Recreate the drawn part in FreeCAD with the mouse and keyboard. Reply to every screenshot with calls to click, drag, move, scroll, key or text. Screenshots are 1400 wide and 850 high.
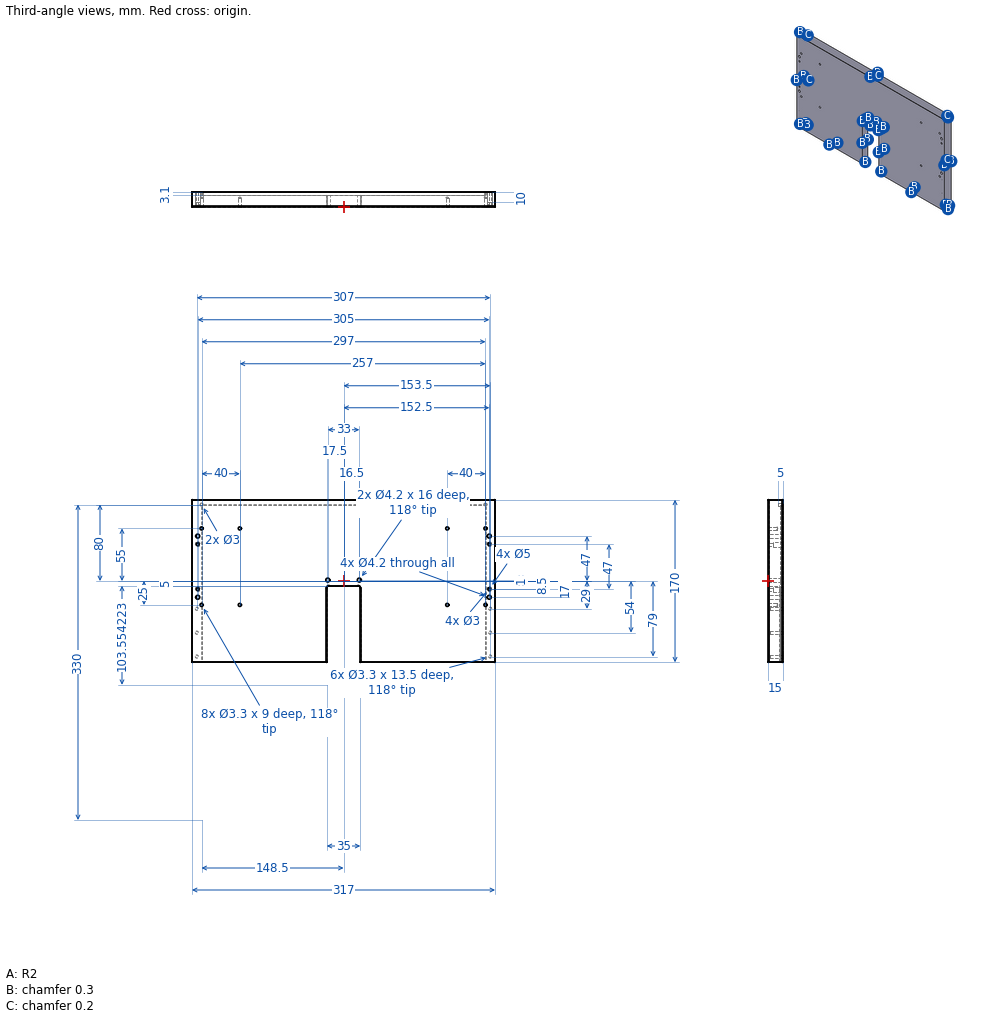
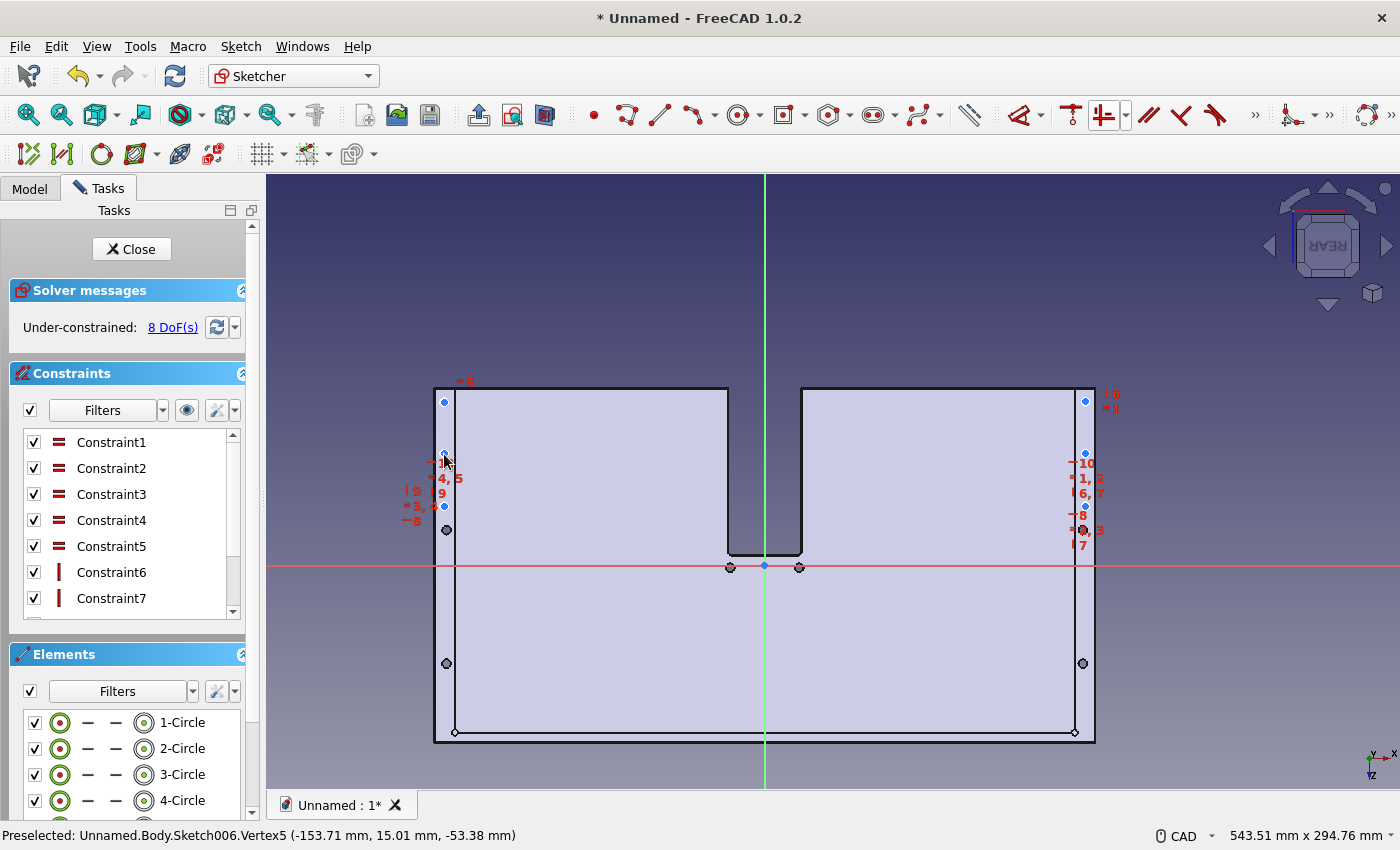
click(444, 453)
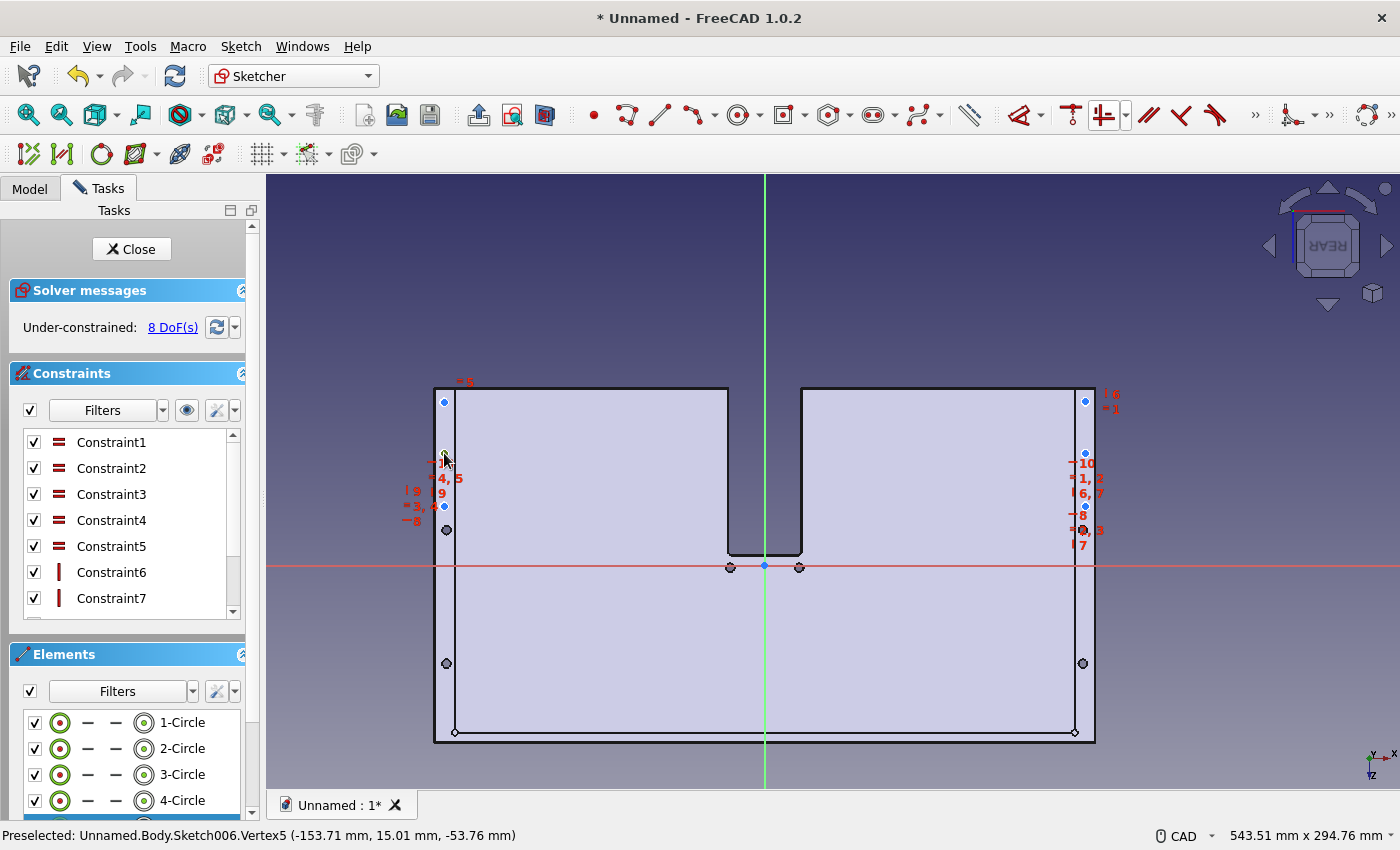
click(444, 402)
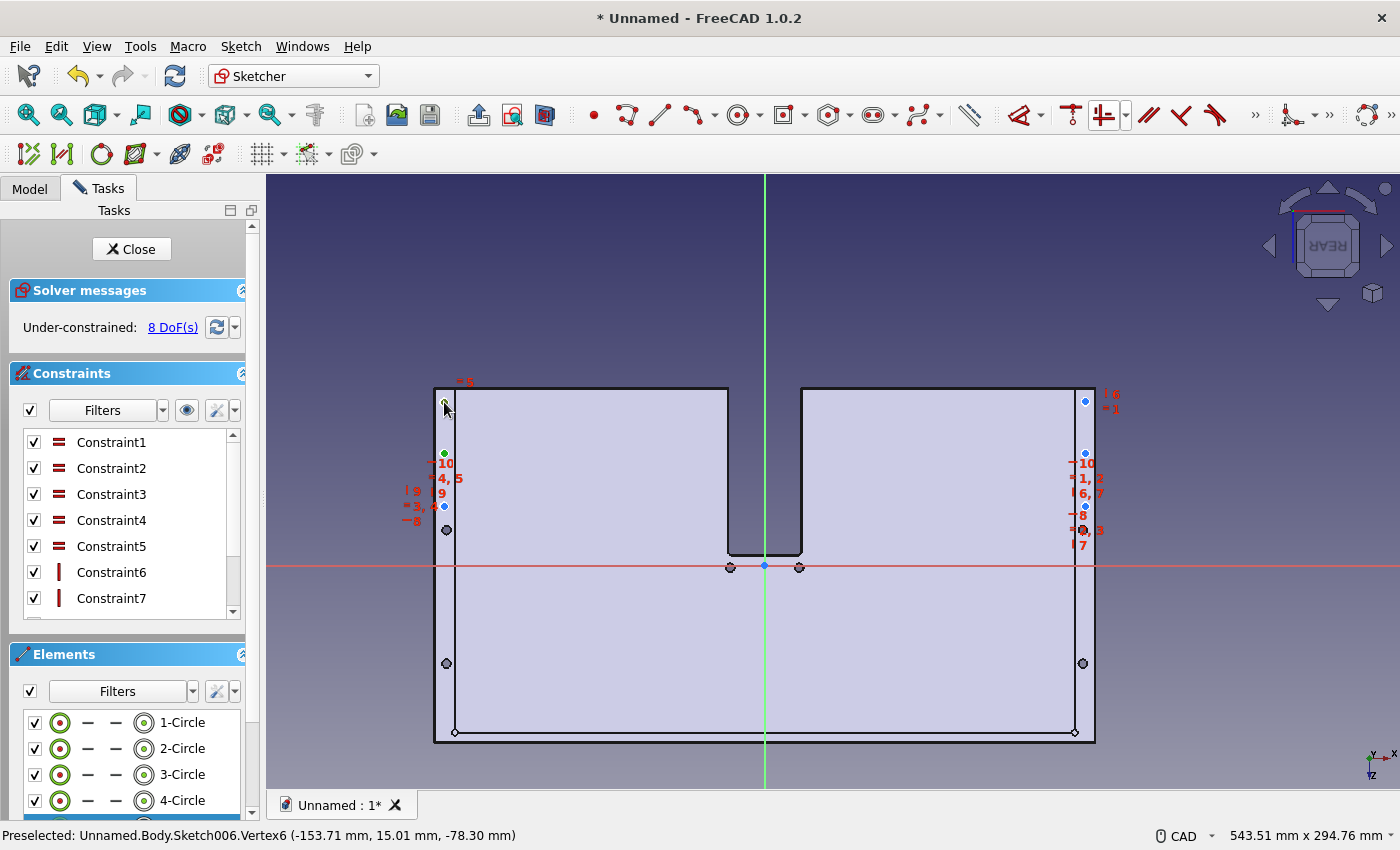
key(v)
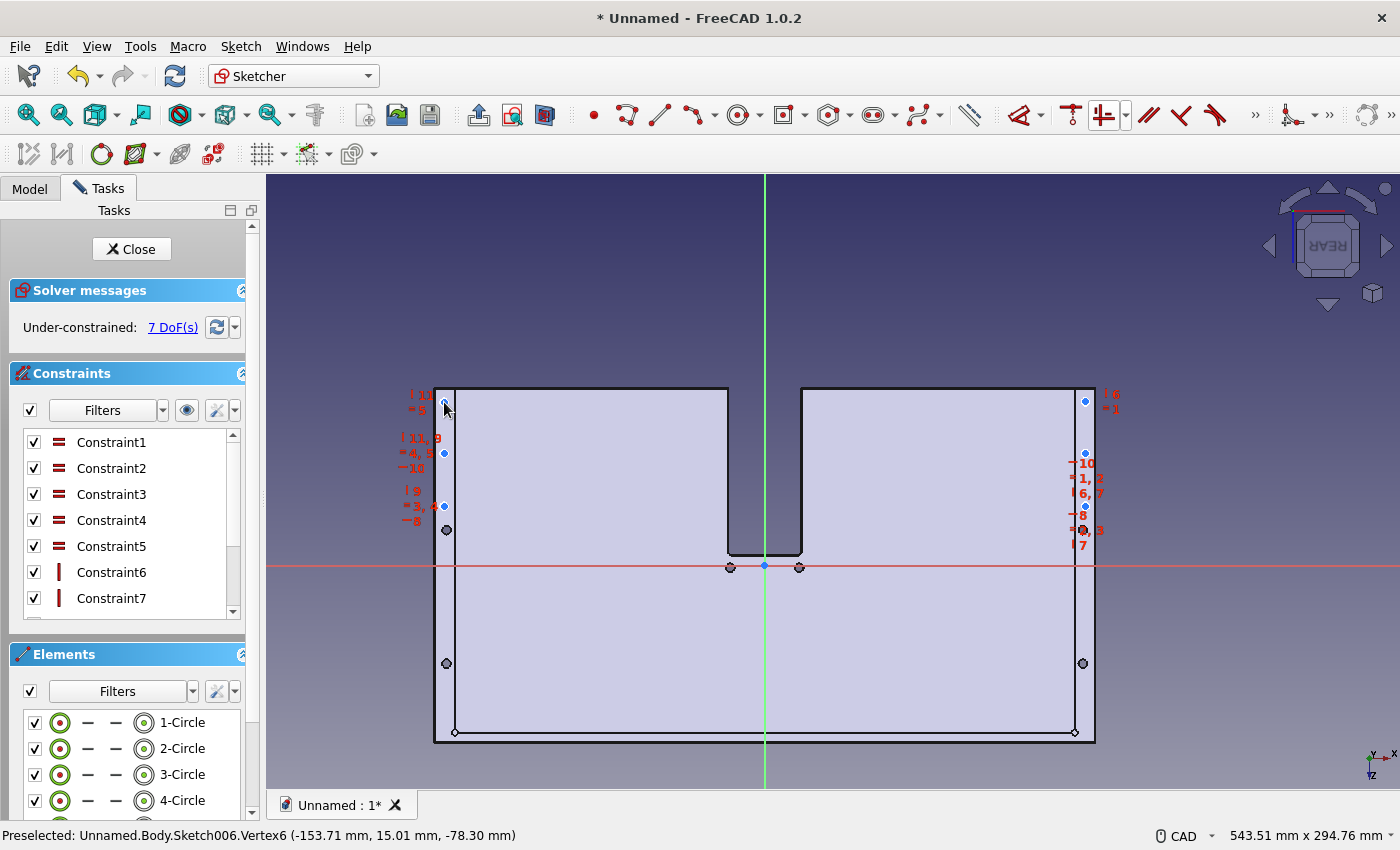
click(1085, 402)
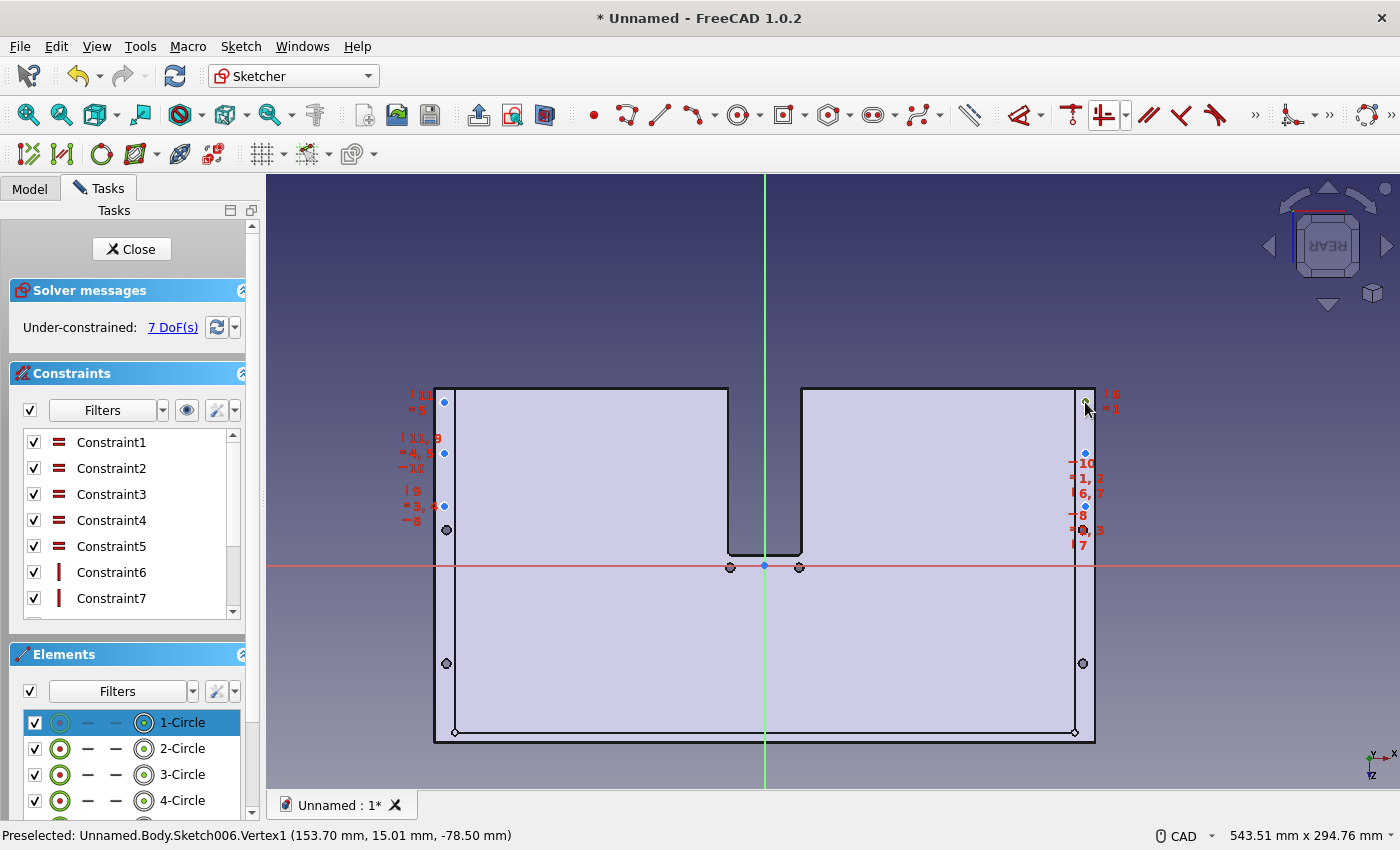
click(444, 402)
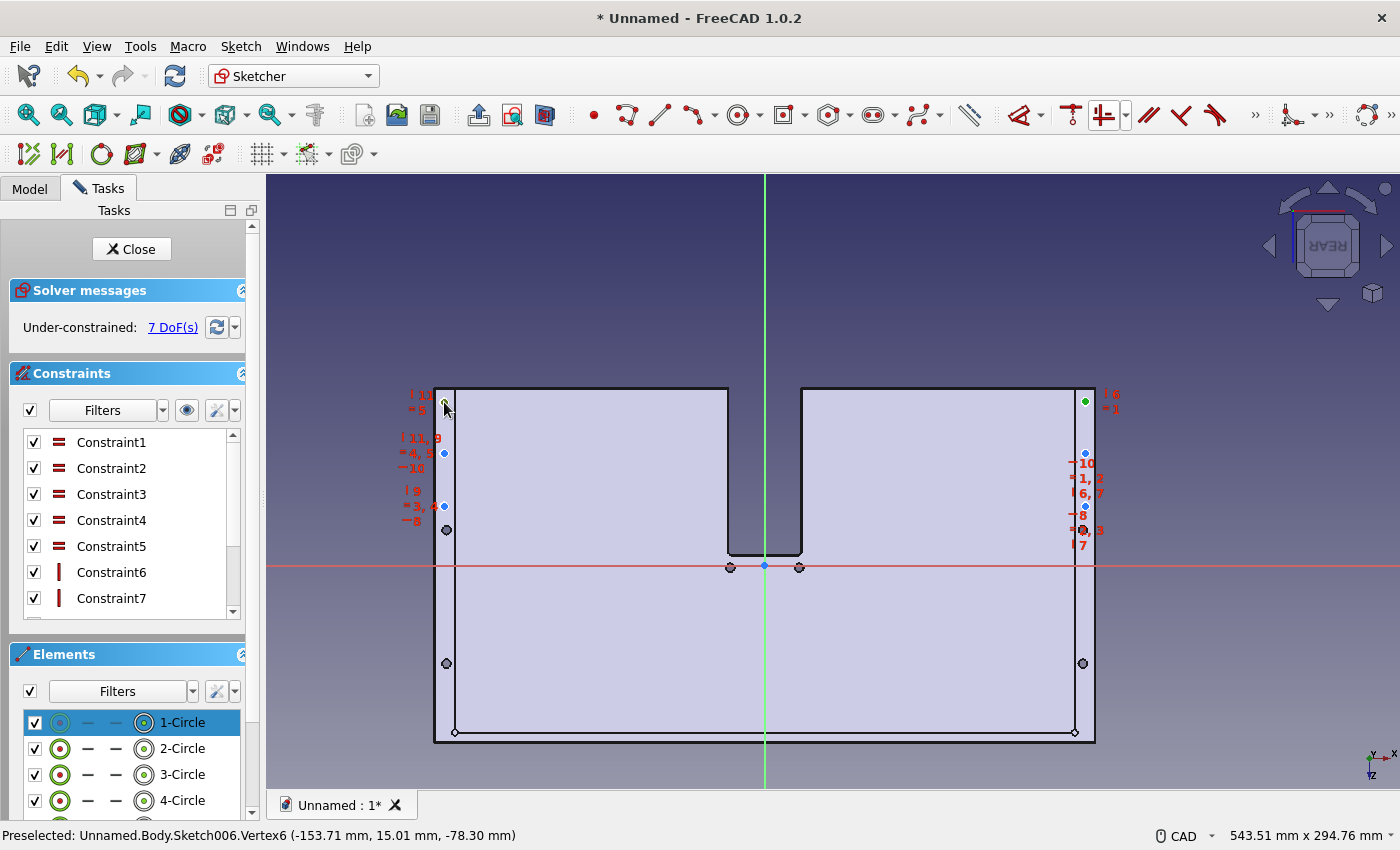
key(h)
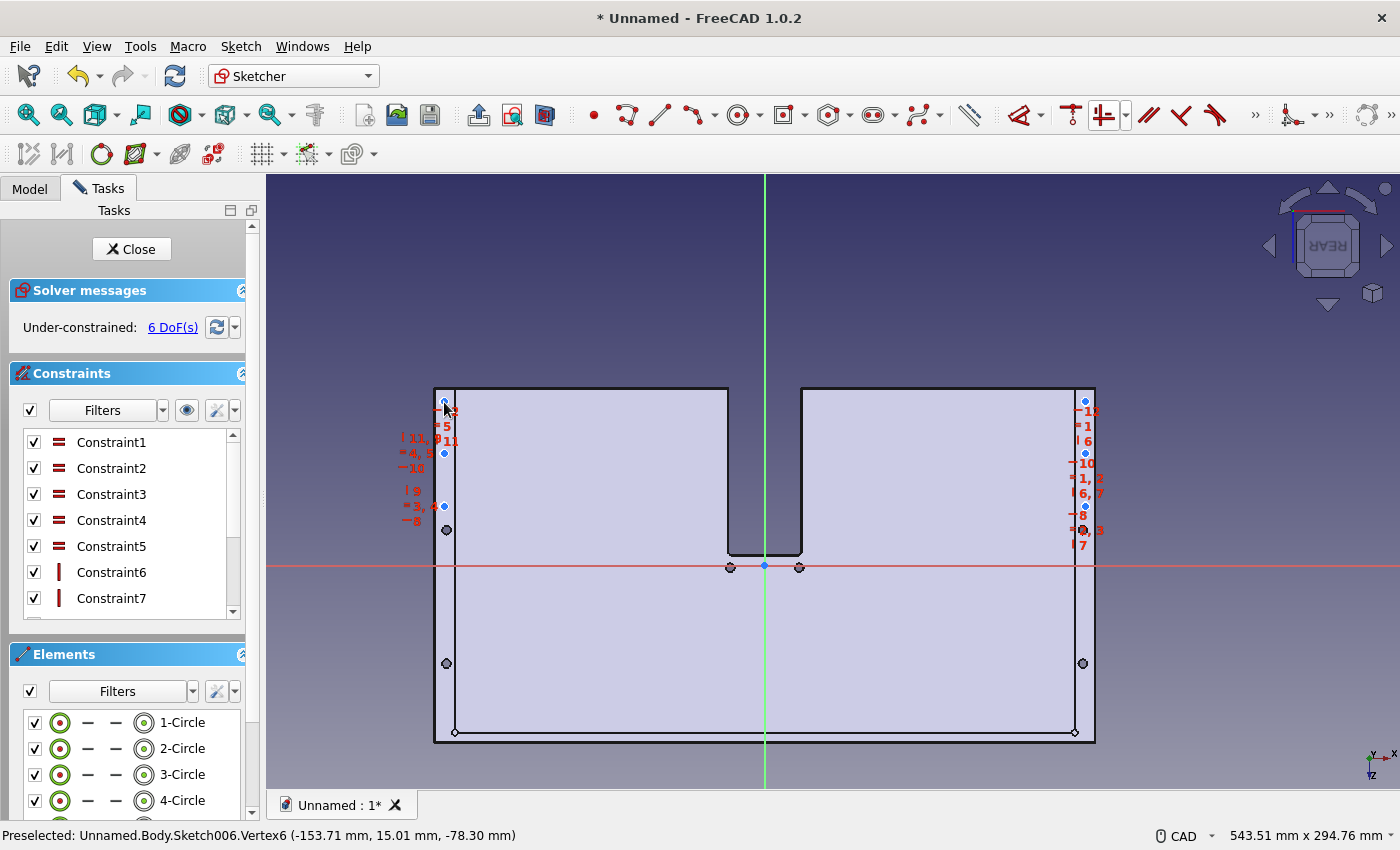
click(1018, 116)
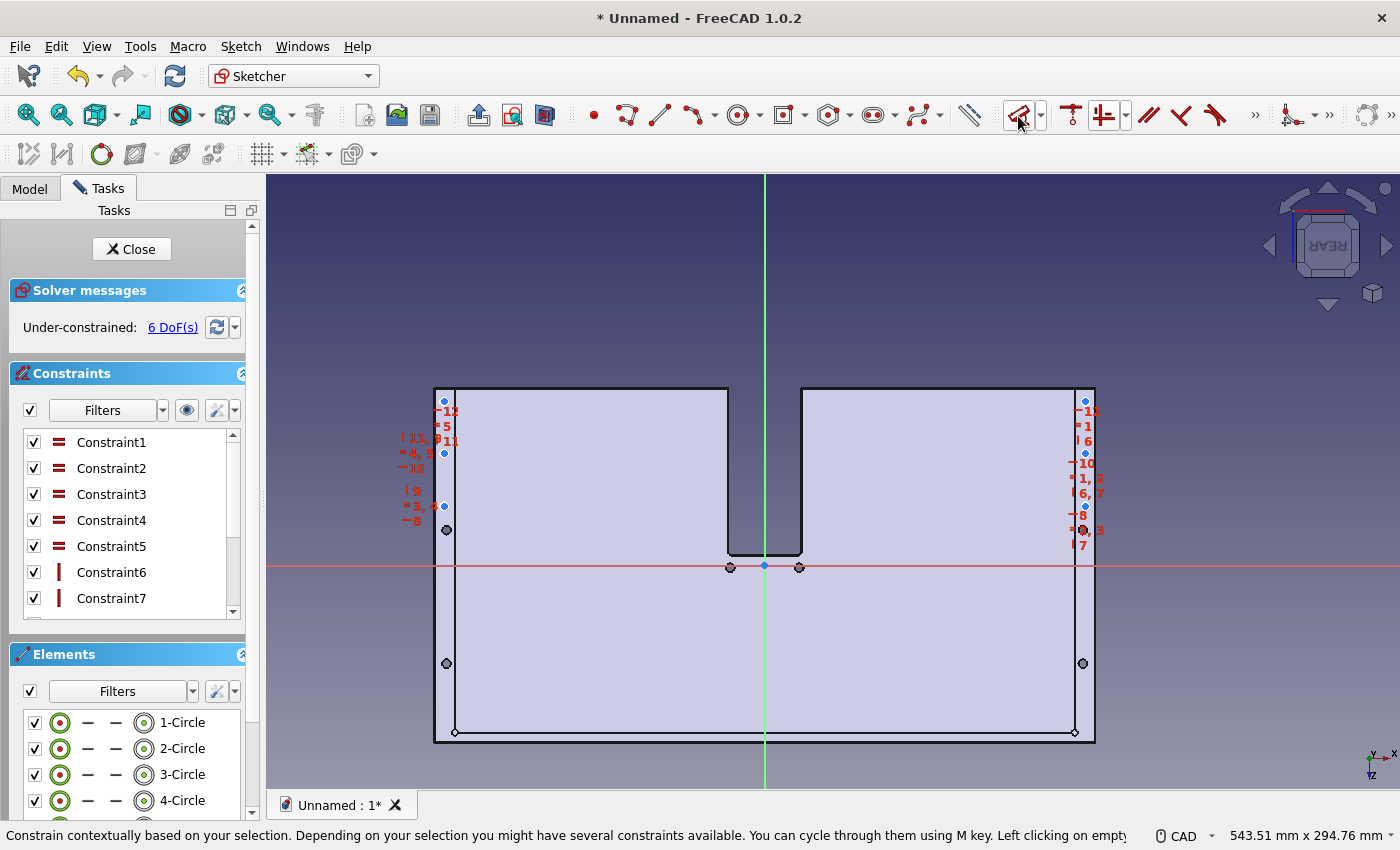
scroll(1086, 398, up, 9)